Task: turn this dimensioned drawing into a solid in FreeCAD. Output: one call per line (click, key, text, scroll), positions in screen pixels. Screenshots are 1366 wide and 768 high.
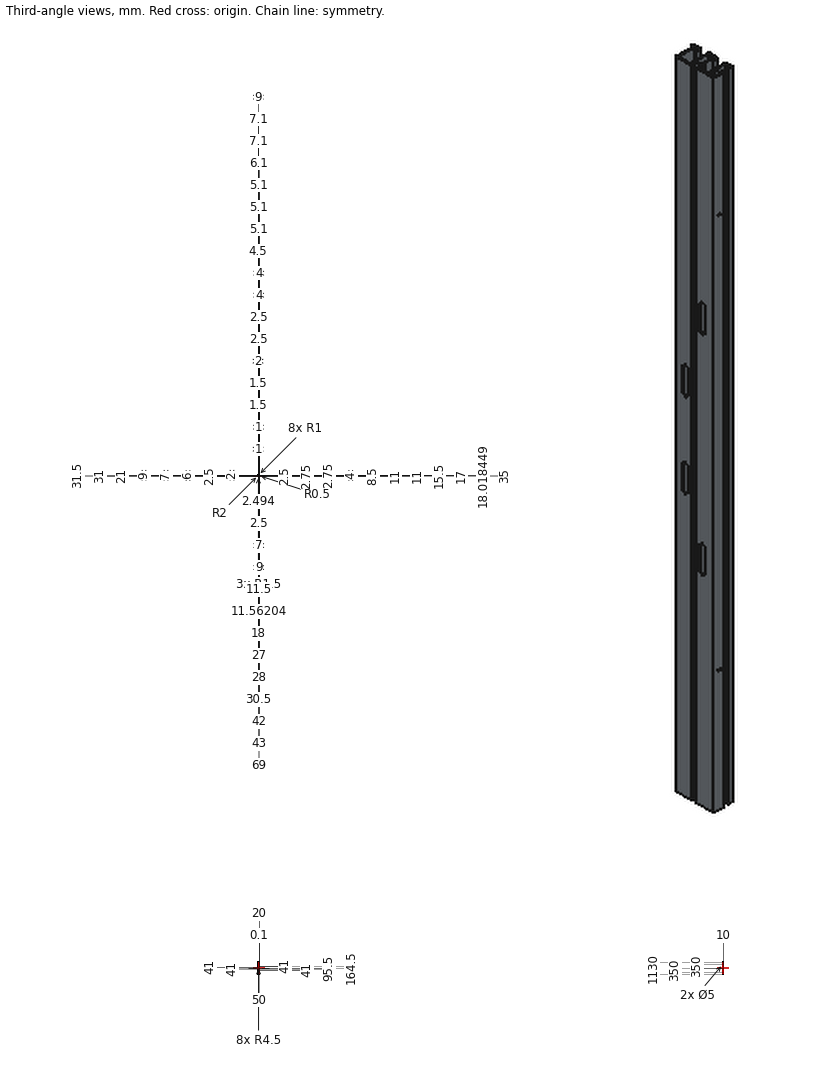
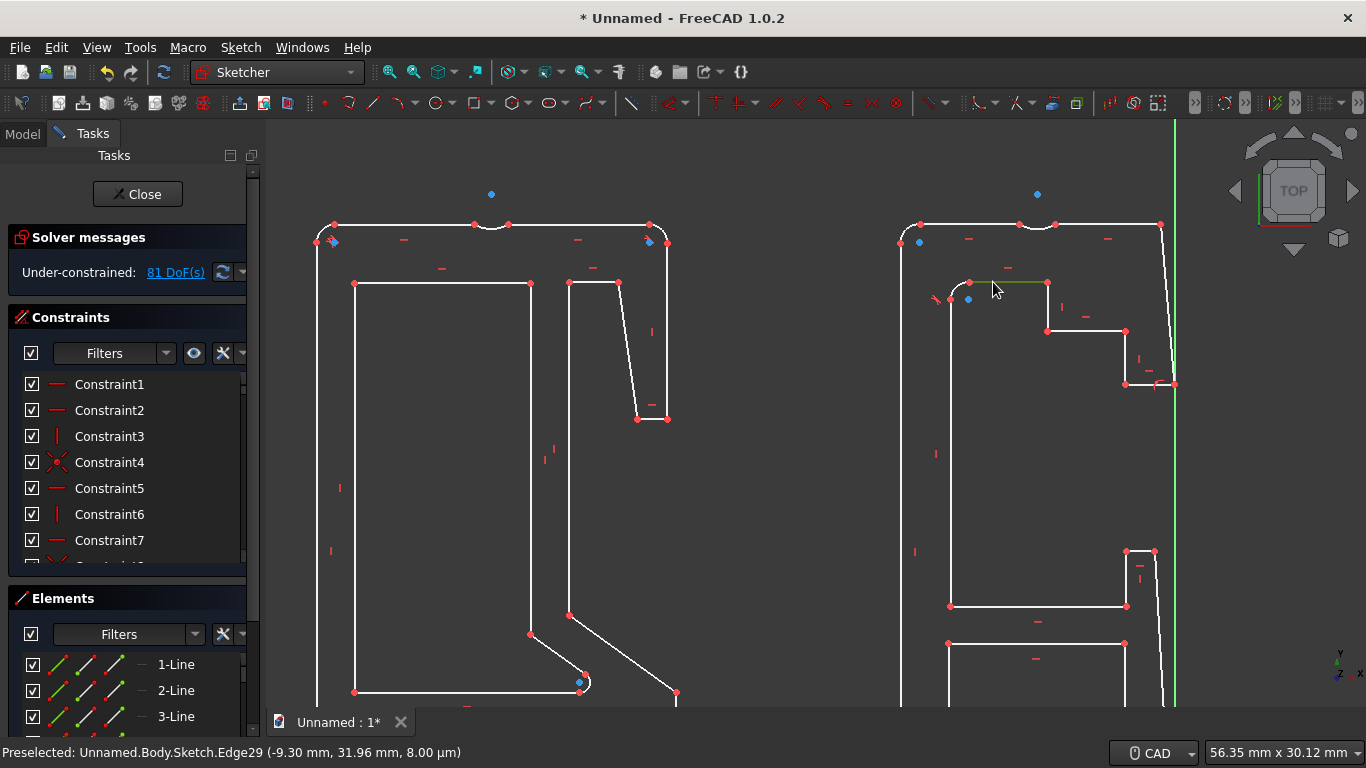
click(956, 287)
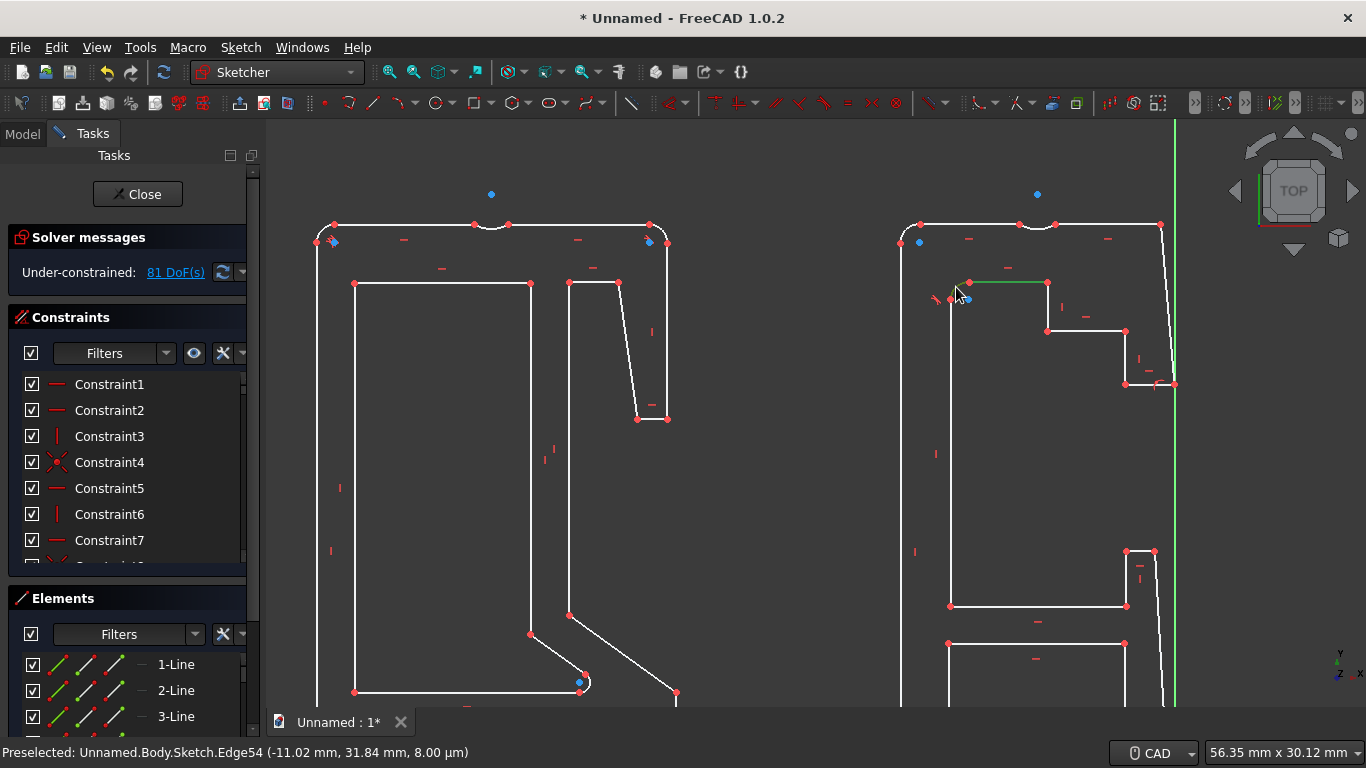
click(824, 104)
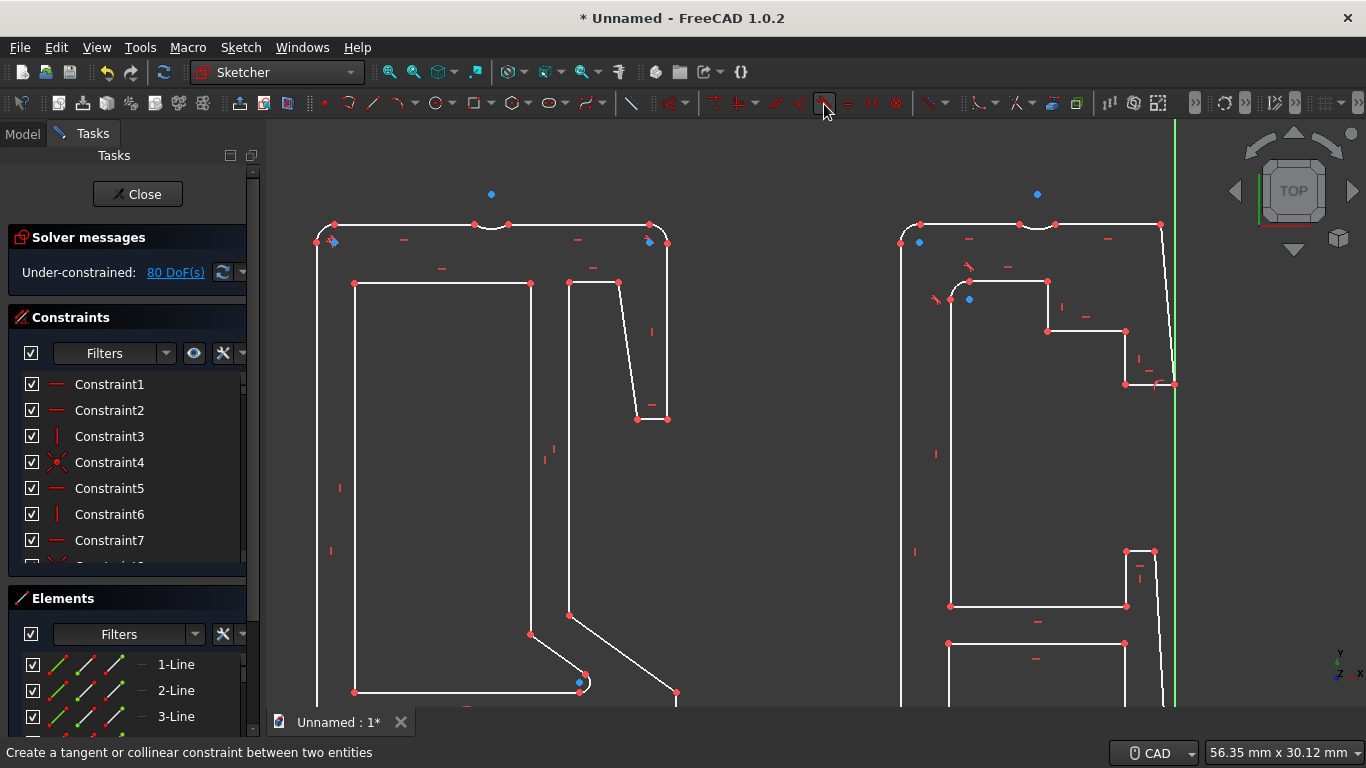
click(990, 224)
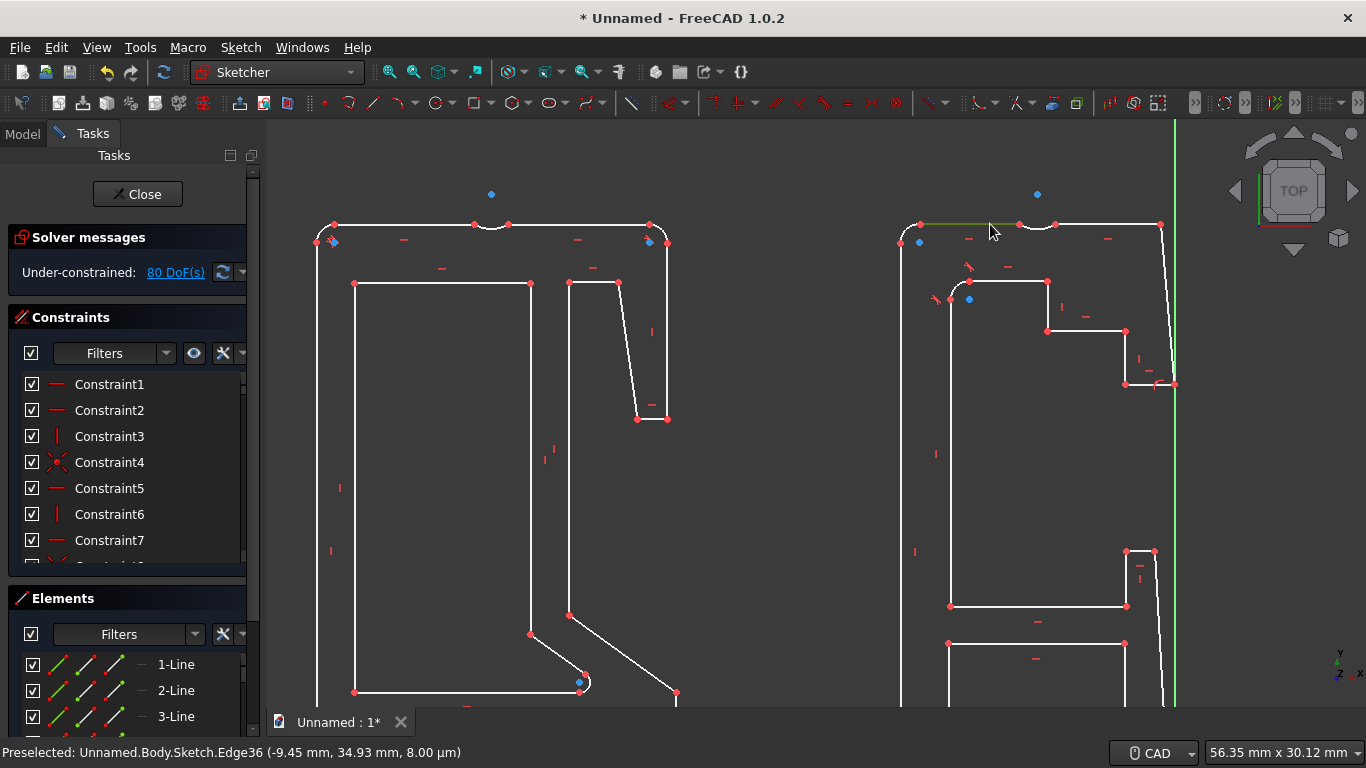
scroll(911, 226, up, 3)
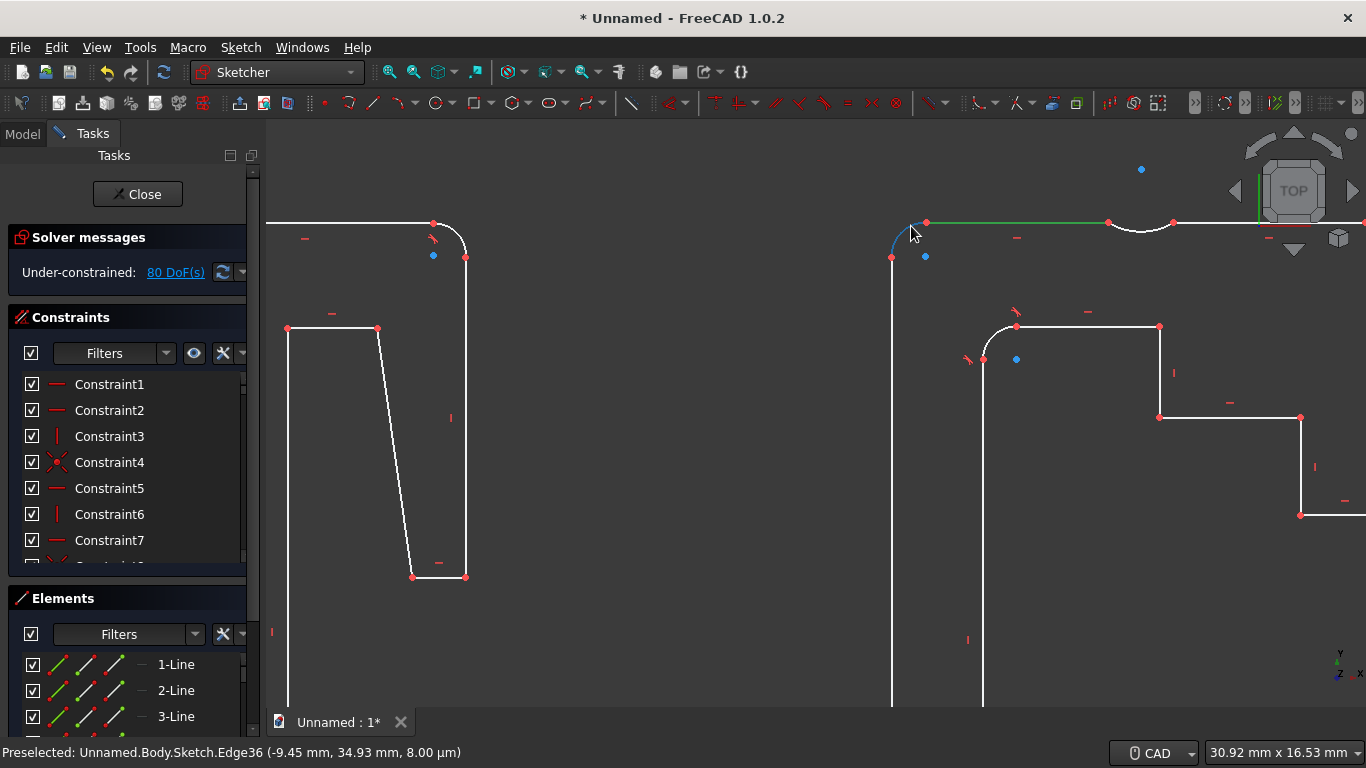
click(911, 226)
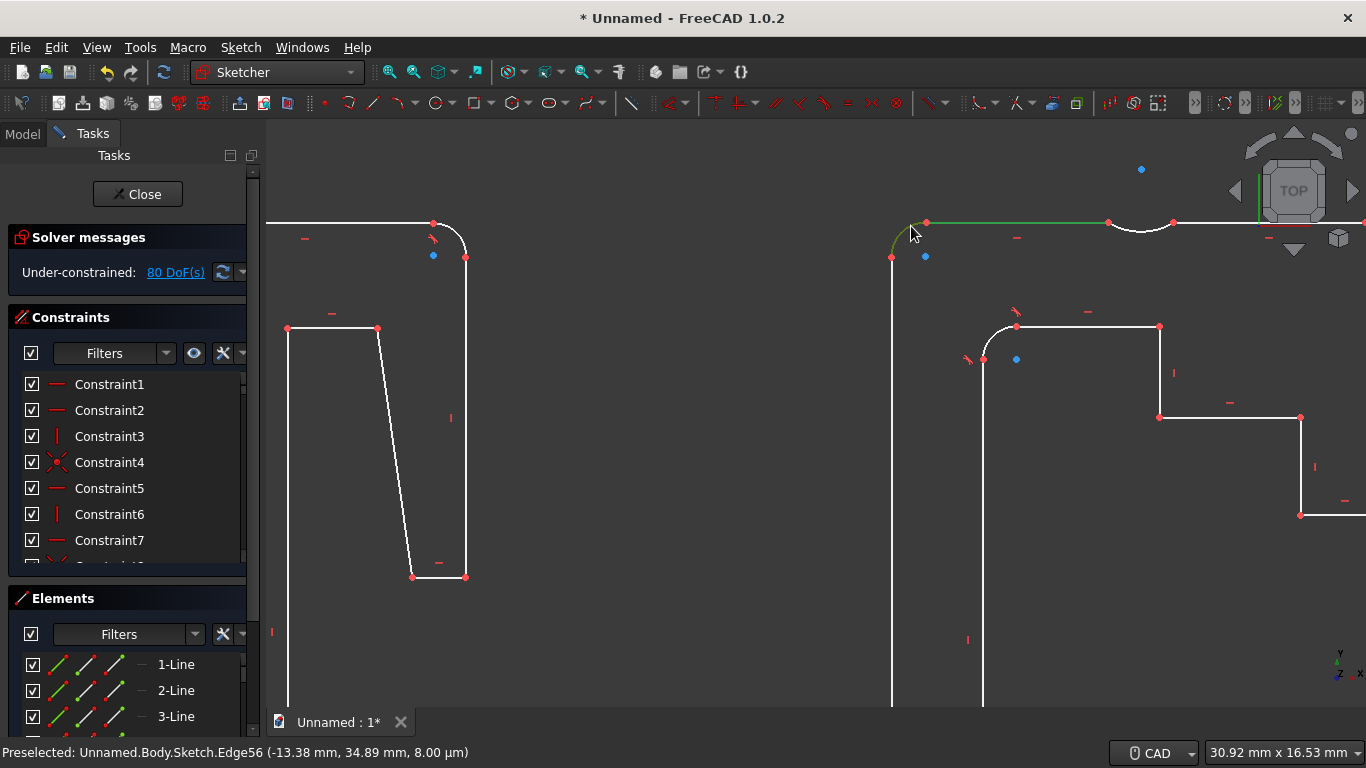
click(824, 104)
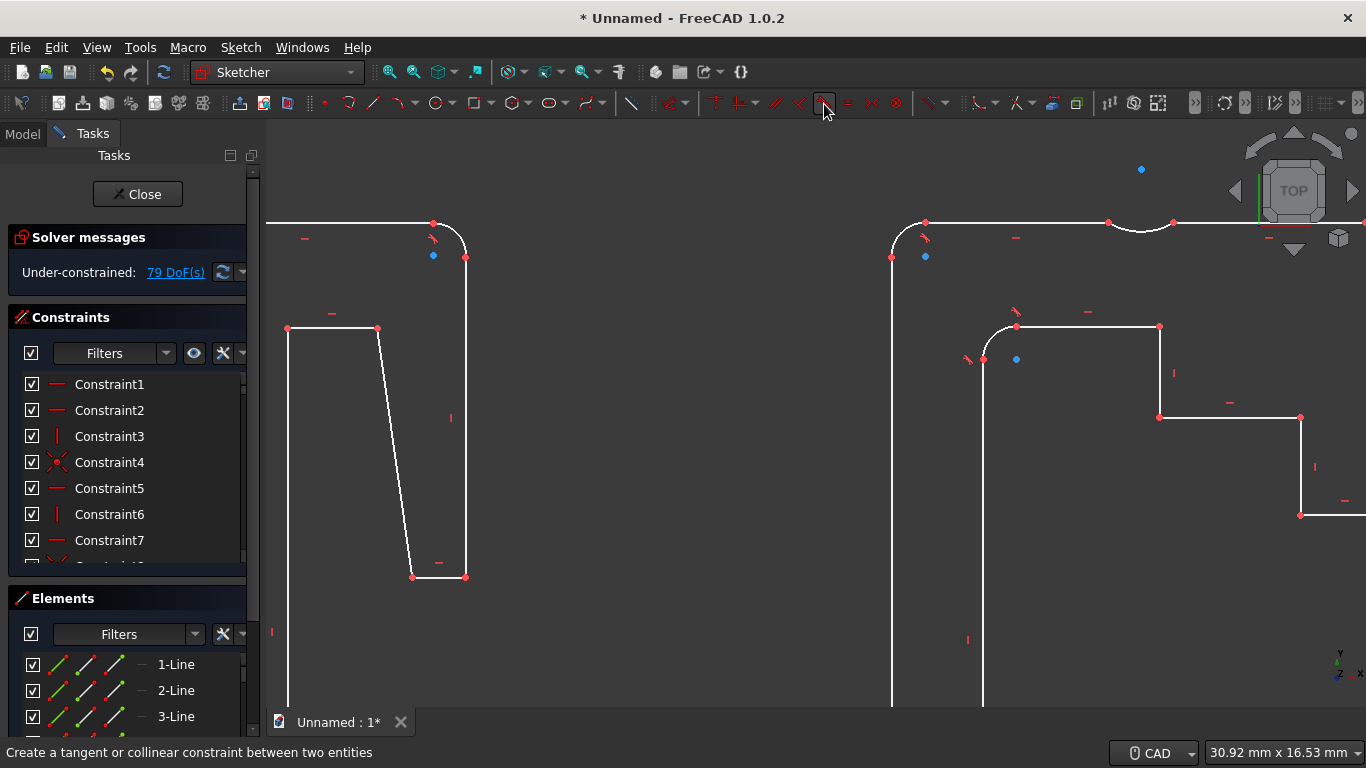
scroll(944, 272, down, 7)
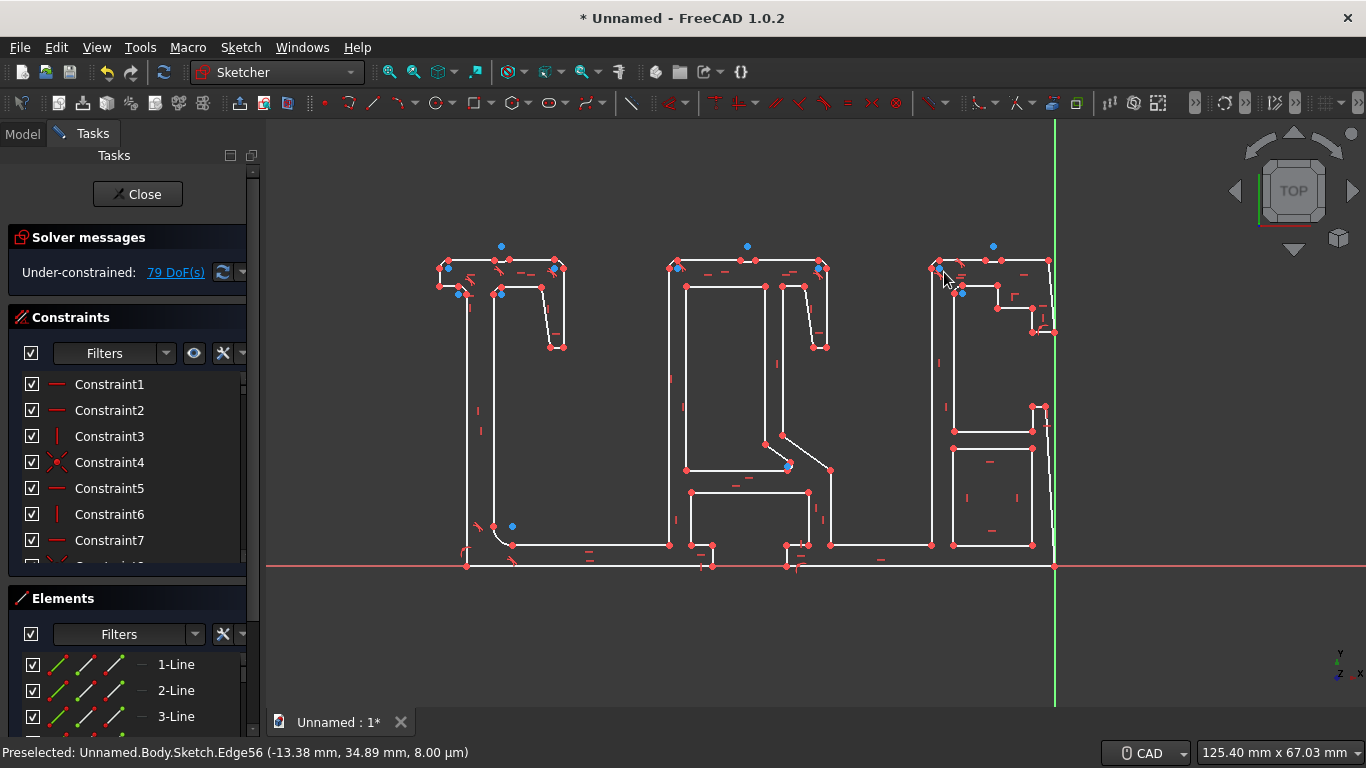
click(932, 352)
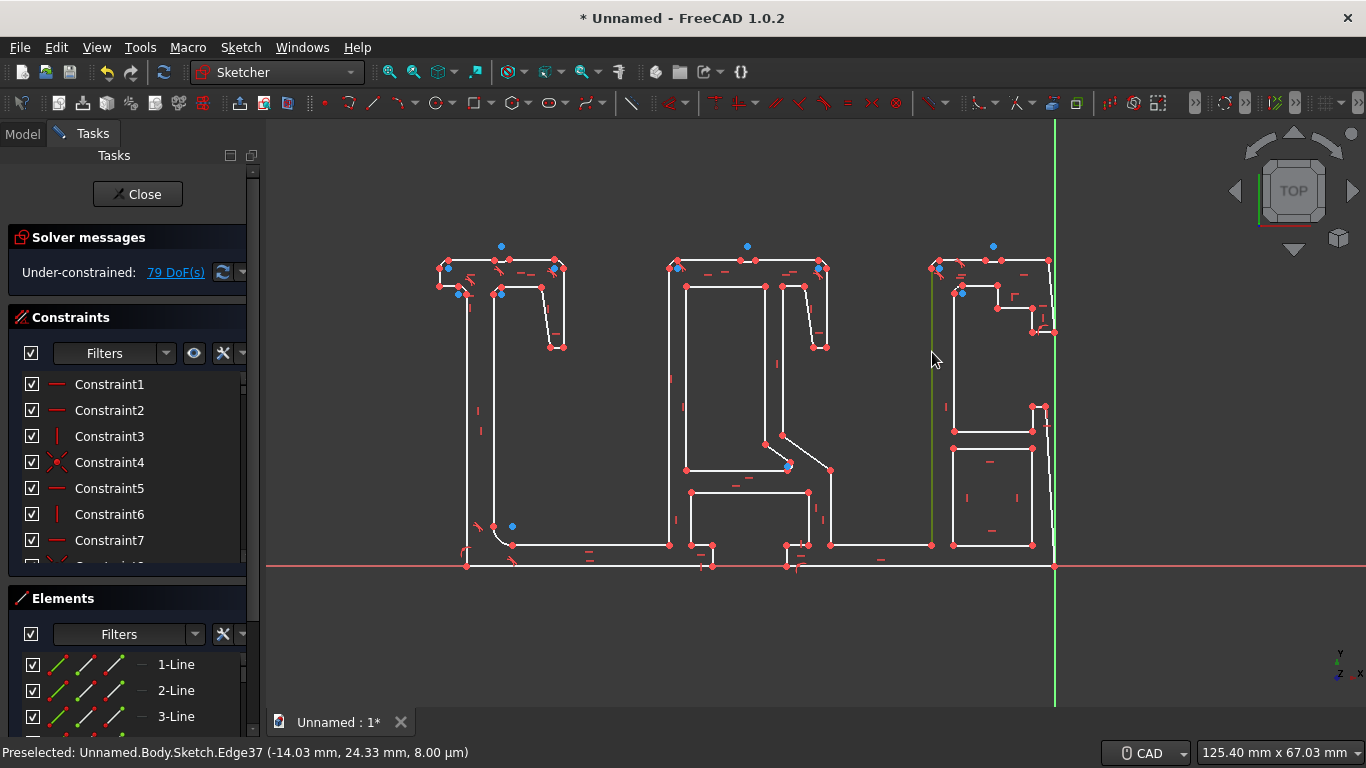
scroll(934, 263, up, 4)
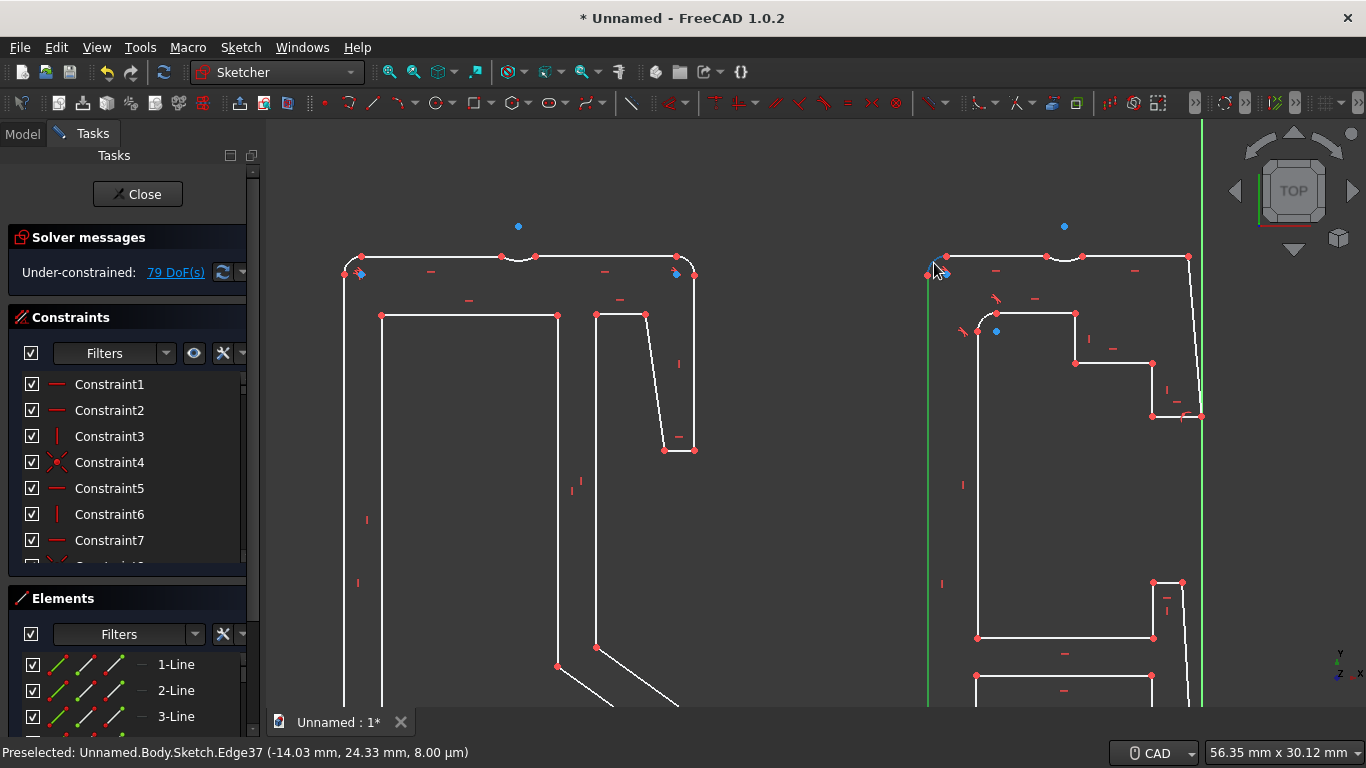
click(933, 262)